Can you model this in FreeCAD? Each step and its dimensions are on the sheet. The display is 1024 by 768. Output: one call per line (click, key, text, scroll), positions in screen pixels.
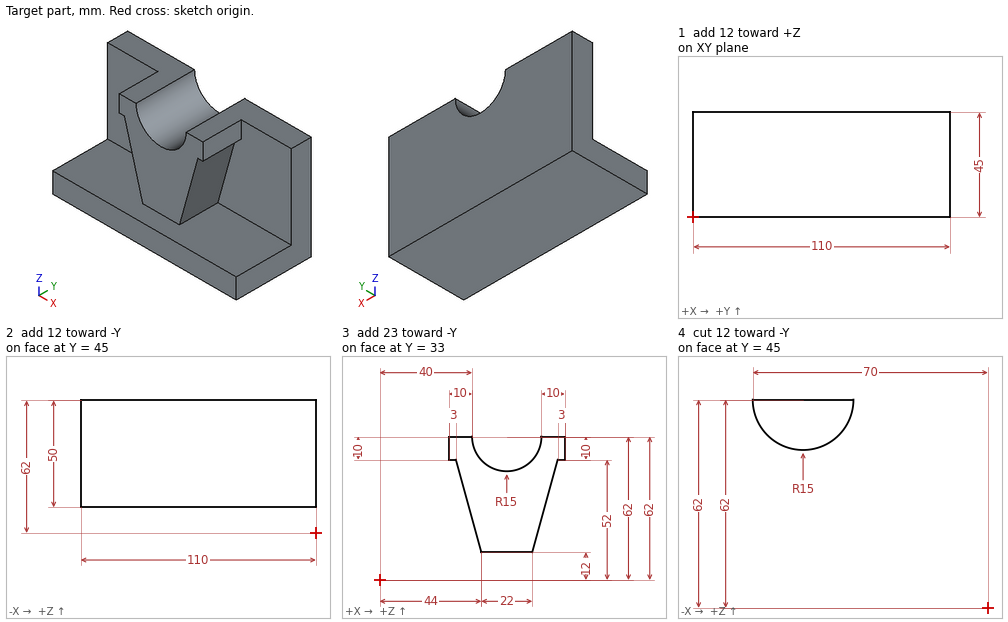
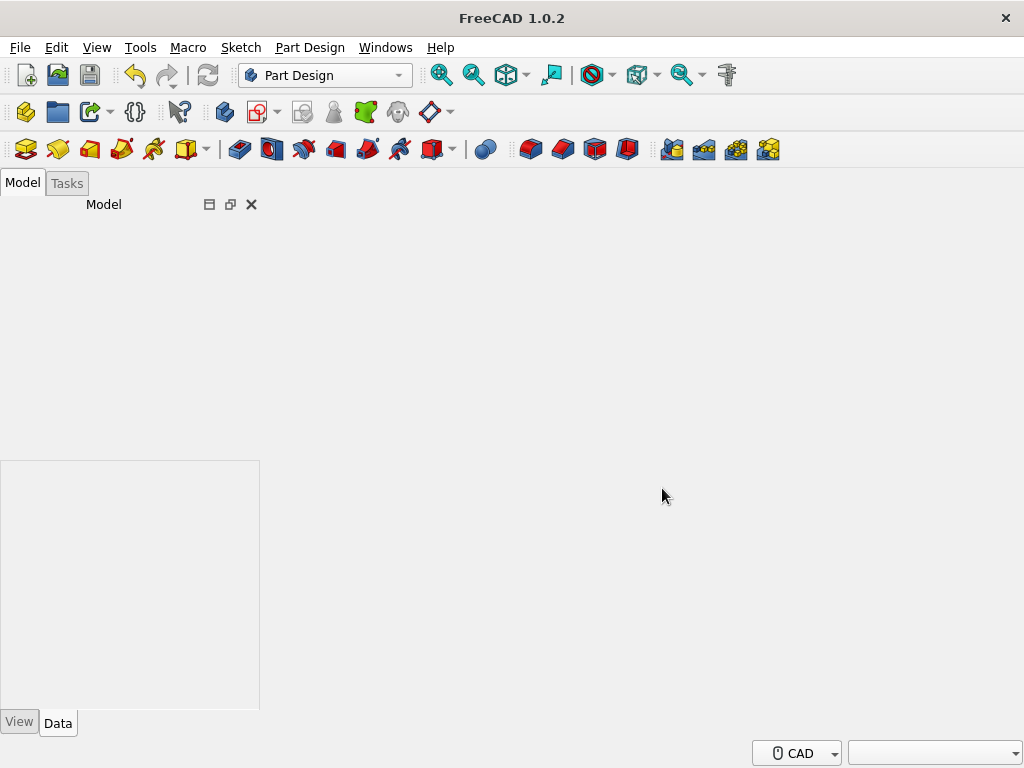
click(26, 76)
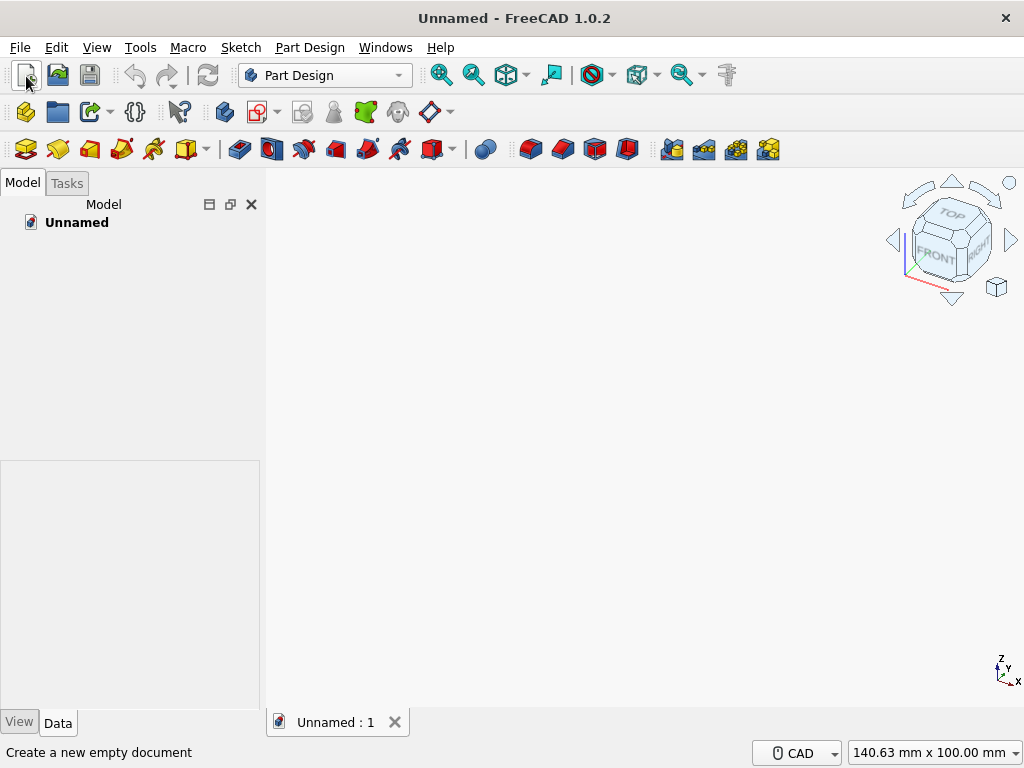
click(258, 112)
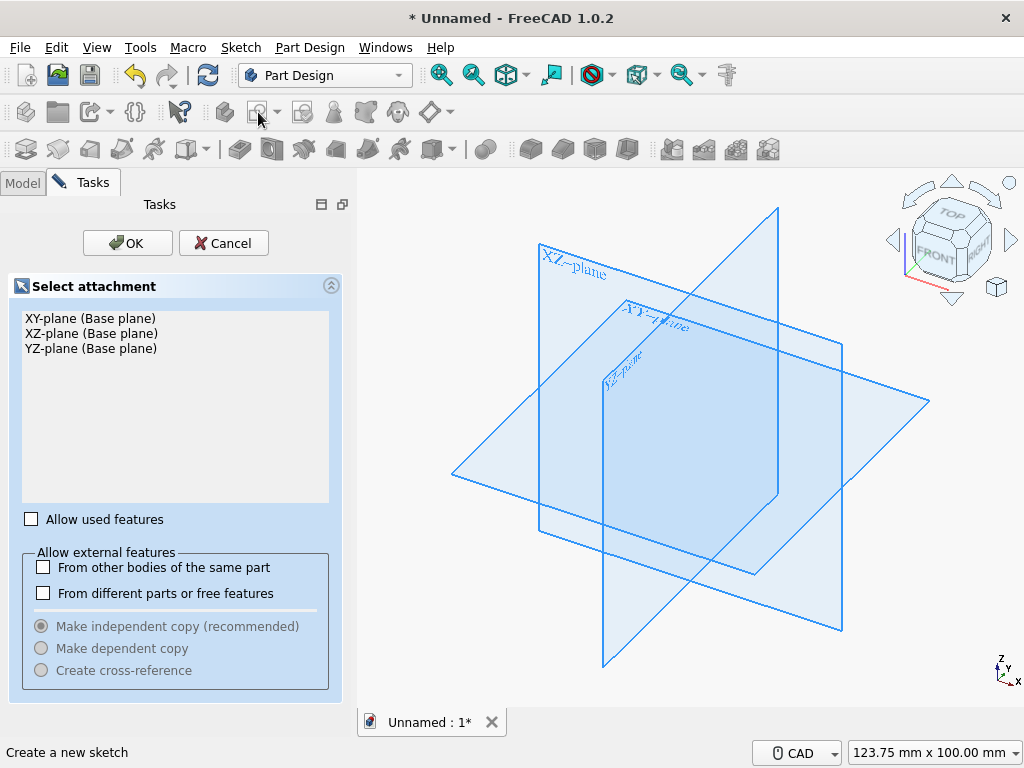
click(82, 318)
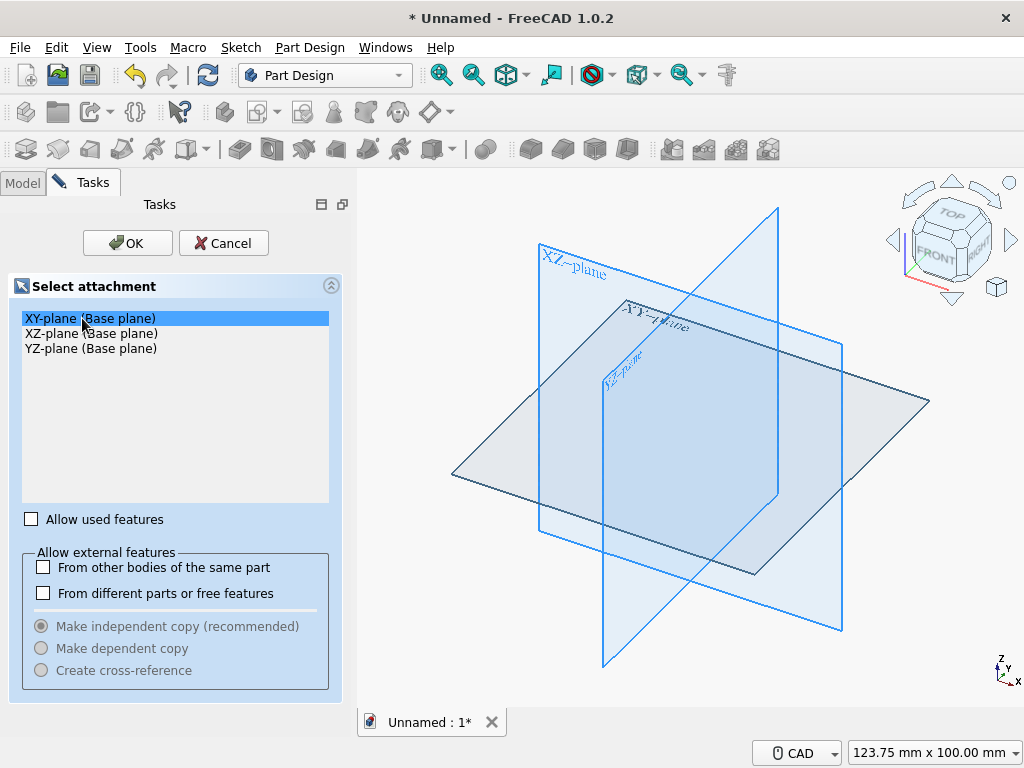
click(128, 243)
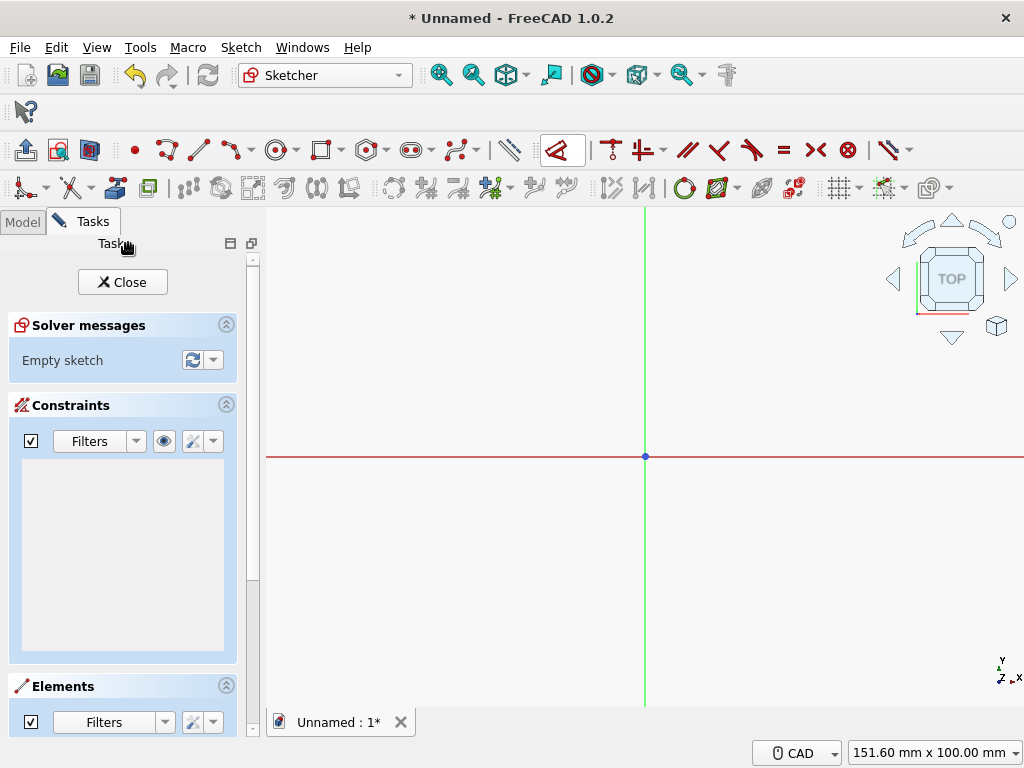
scroll(294, 594, down, 3)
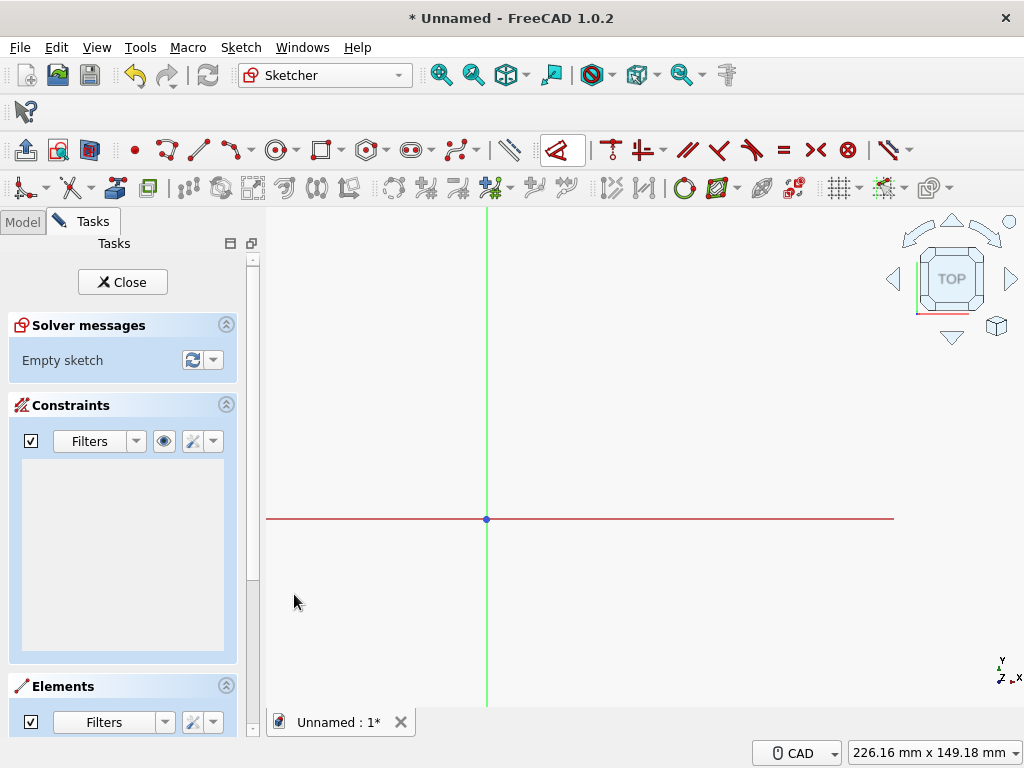
click(322, 150)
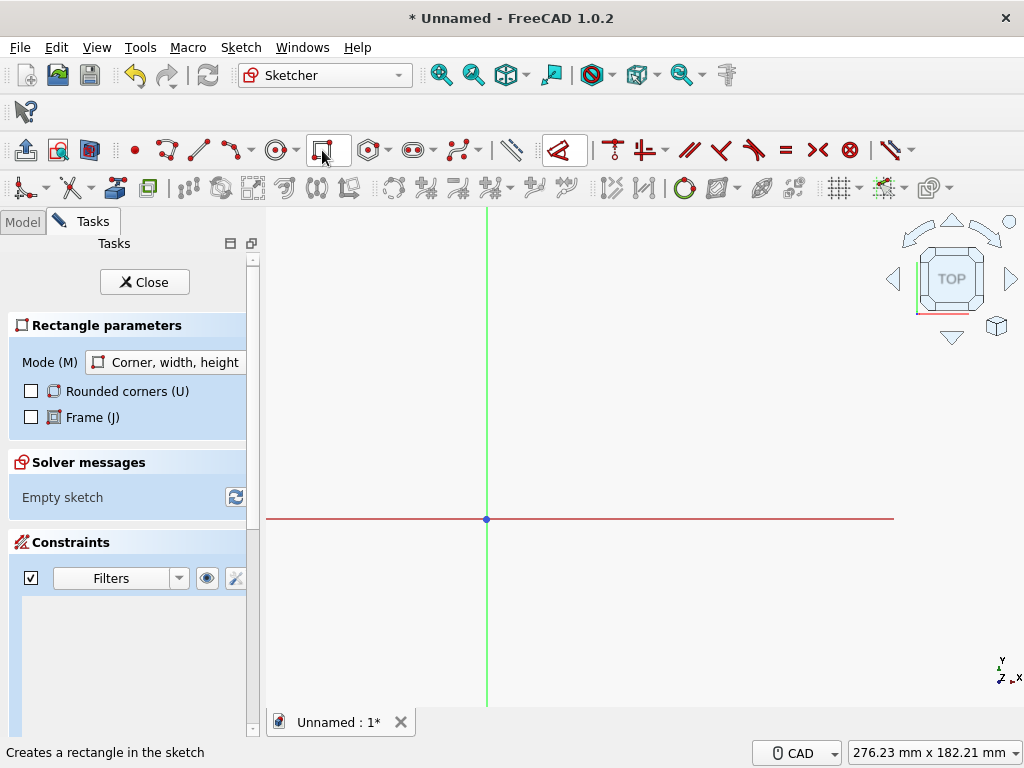
click(487, 519)
move(788, 396)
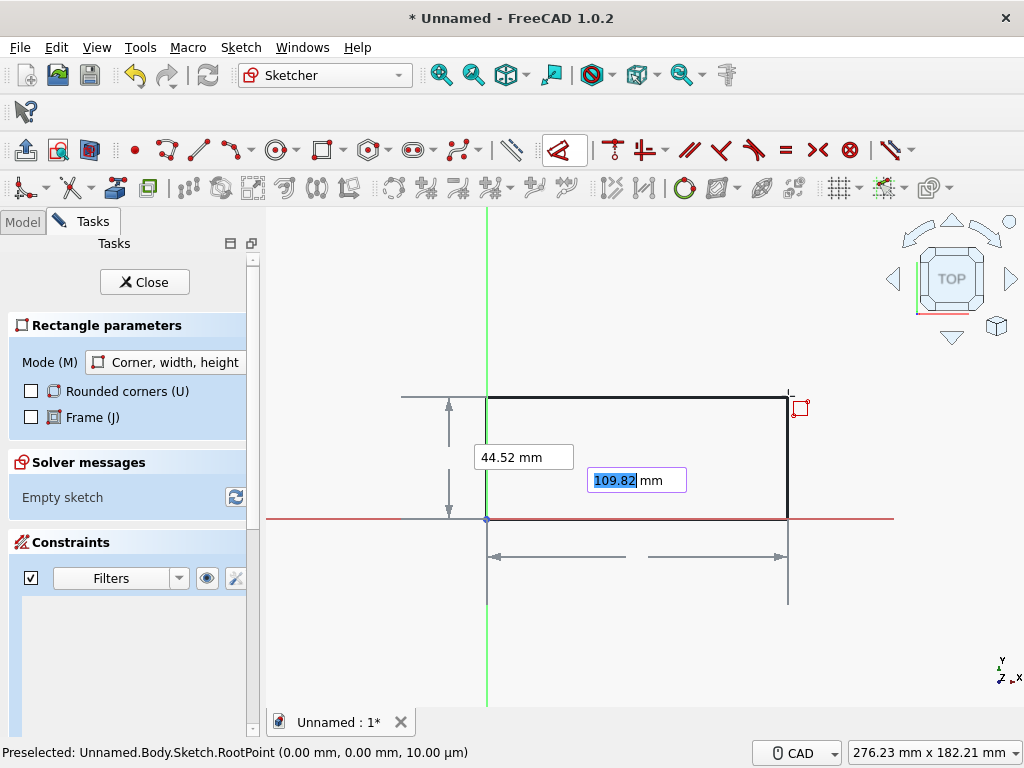
text(110)
key(Tab)
text(45)
key(Return)
key(Escape)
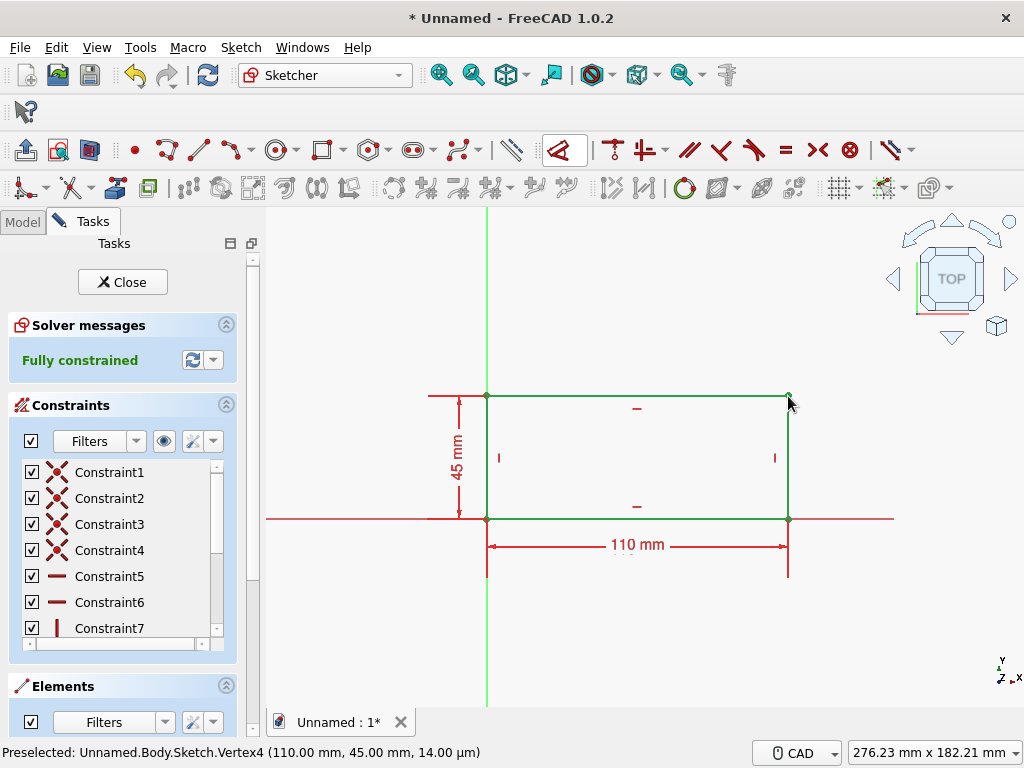
click(123, 282)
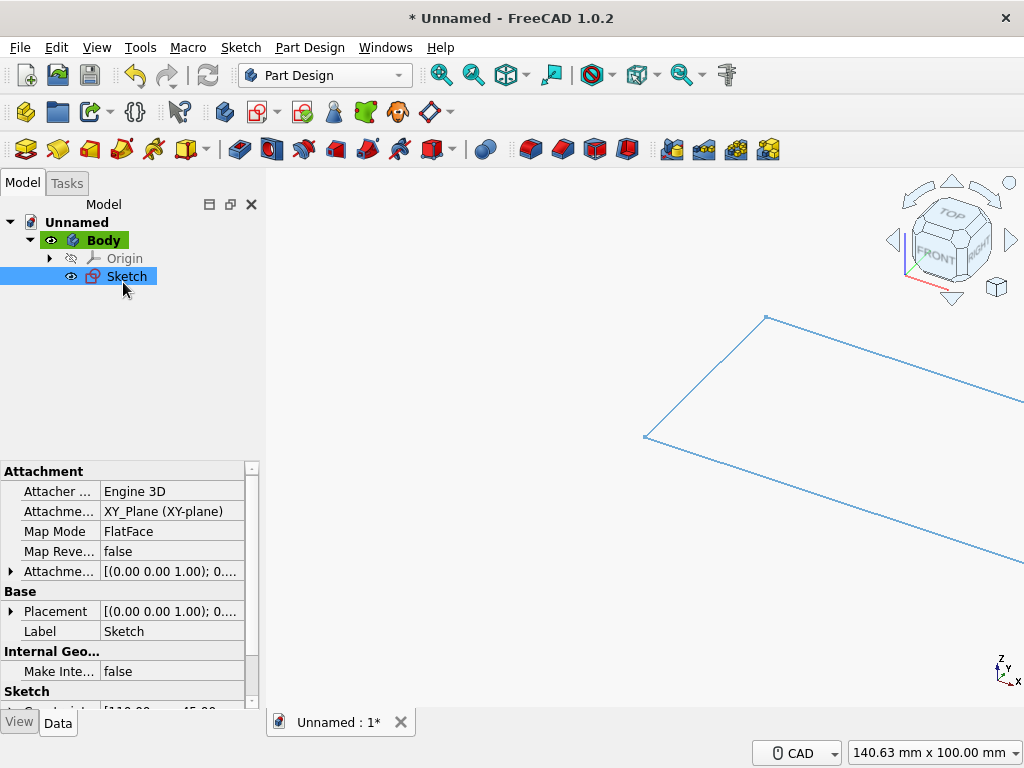
click(26, 150)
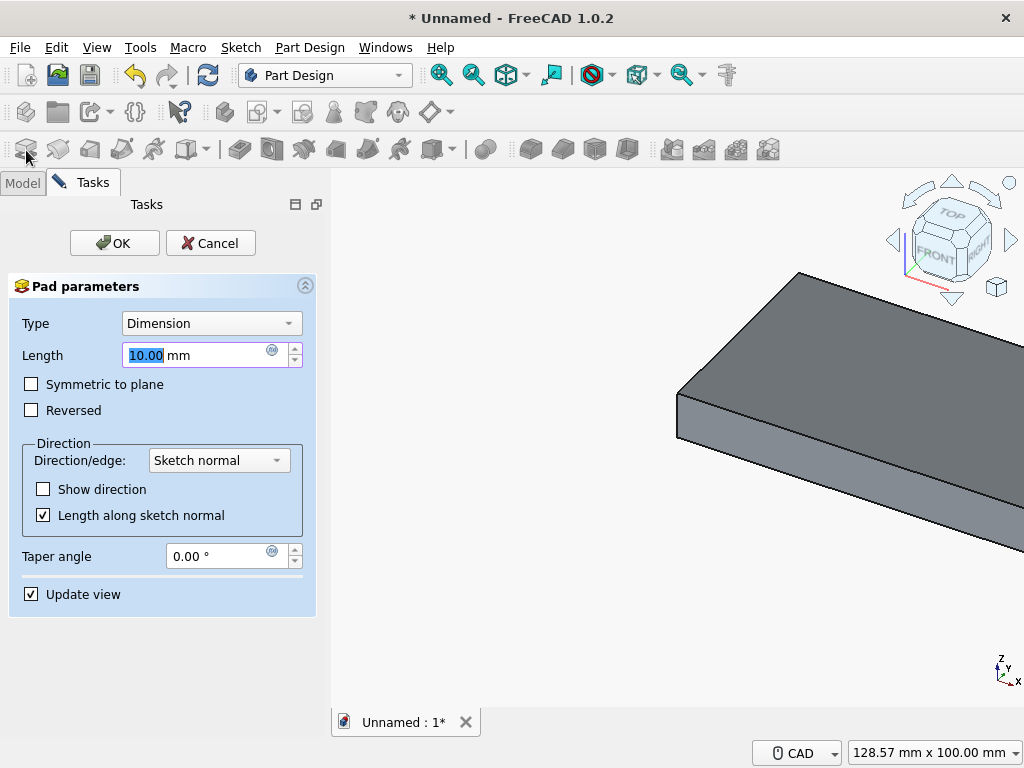
text(12)
key(Tab)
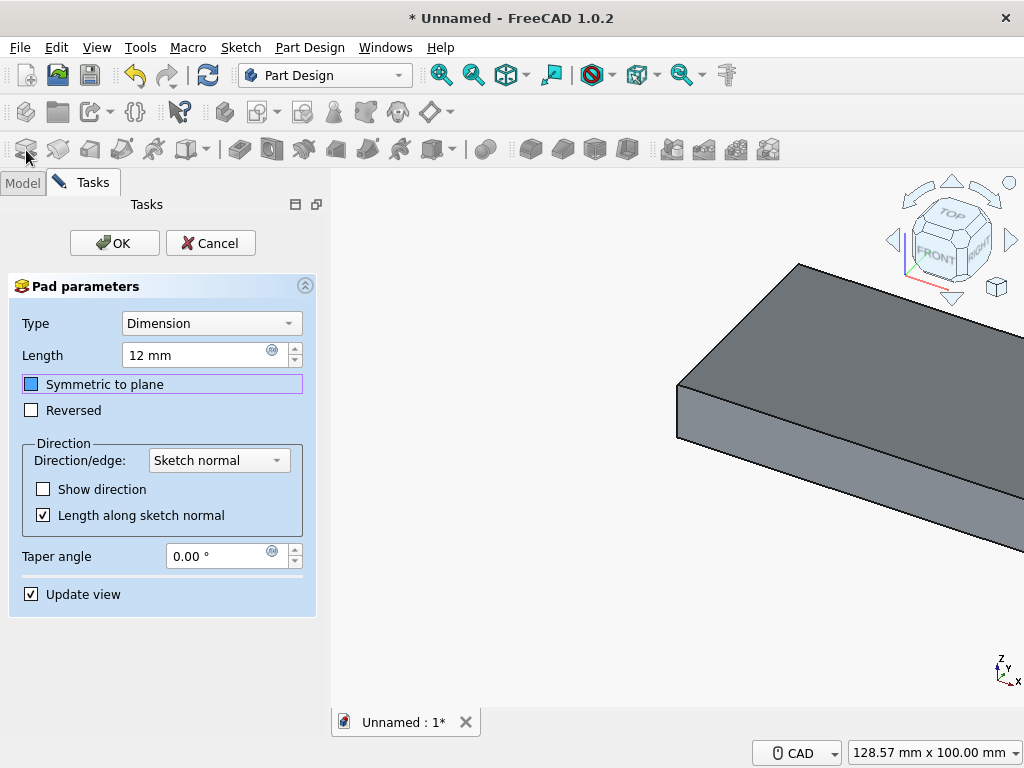
click(115, 243)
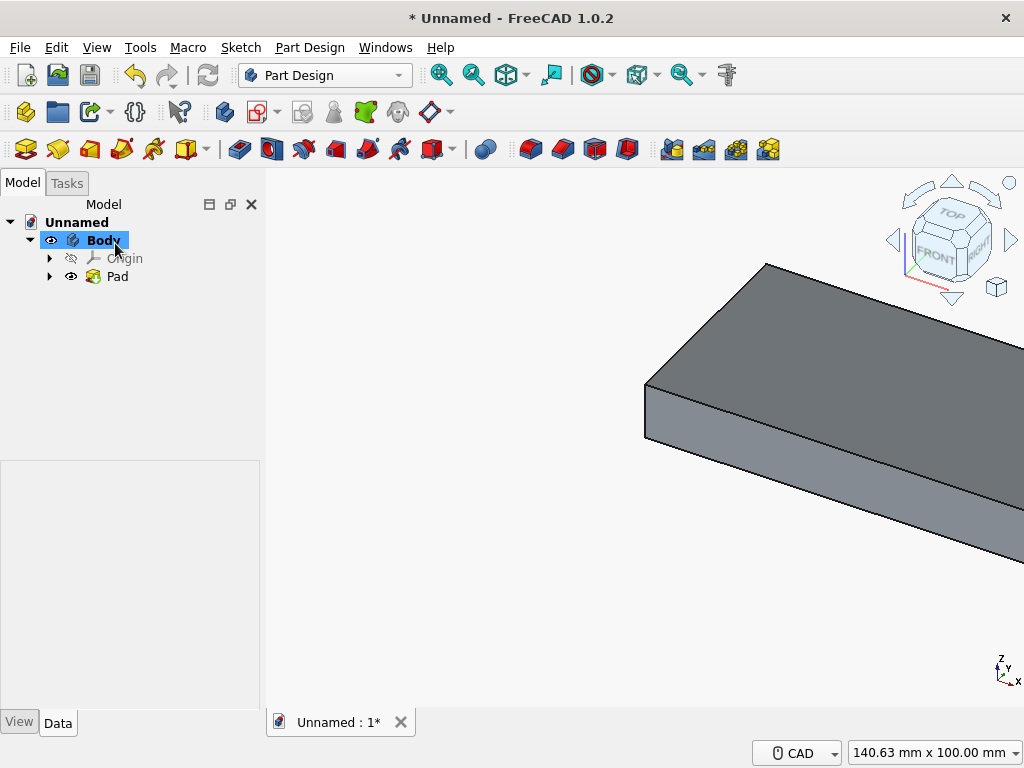
click(442, 76)